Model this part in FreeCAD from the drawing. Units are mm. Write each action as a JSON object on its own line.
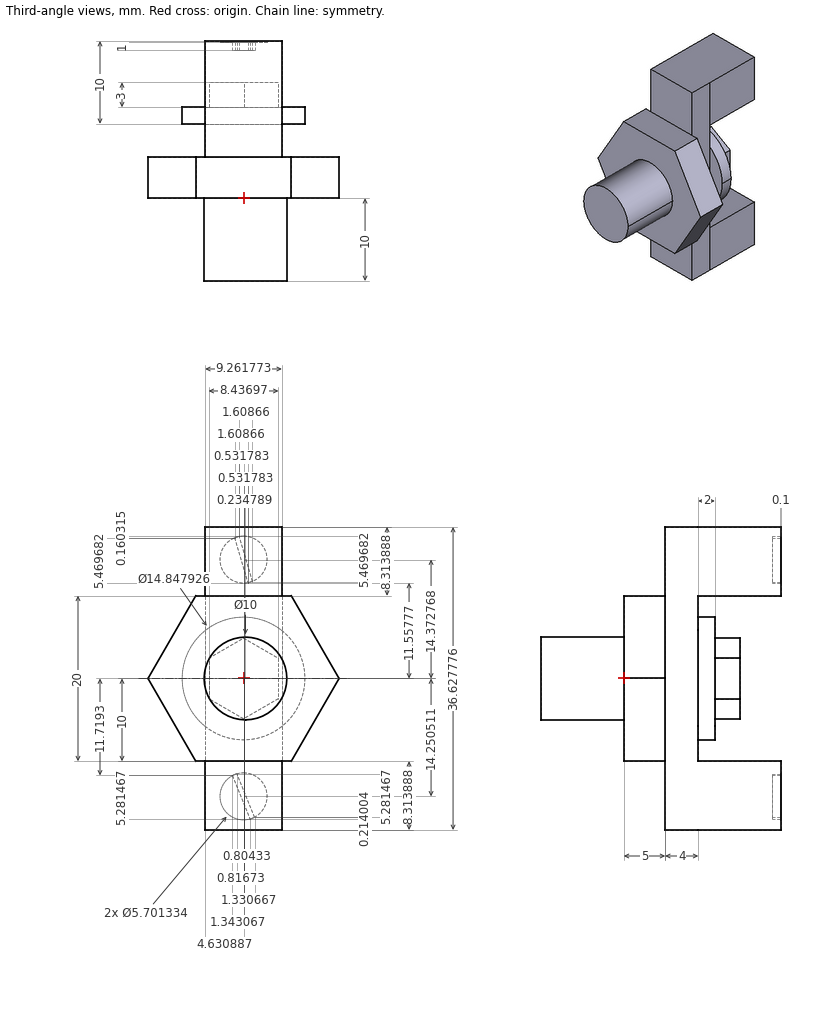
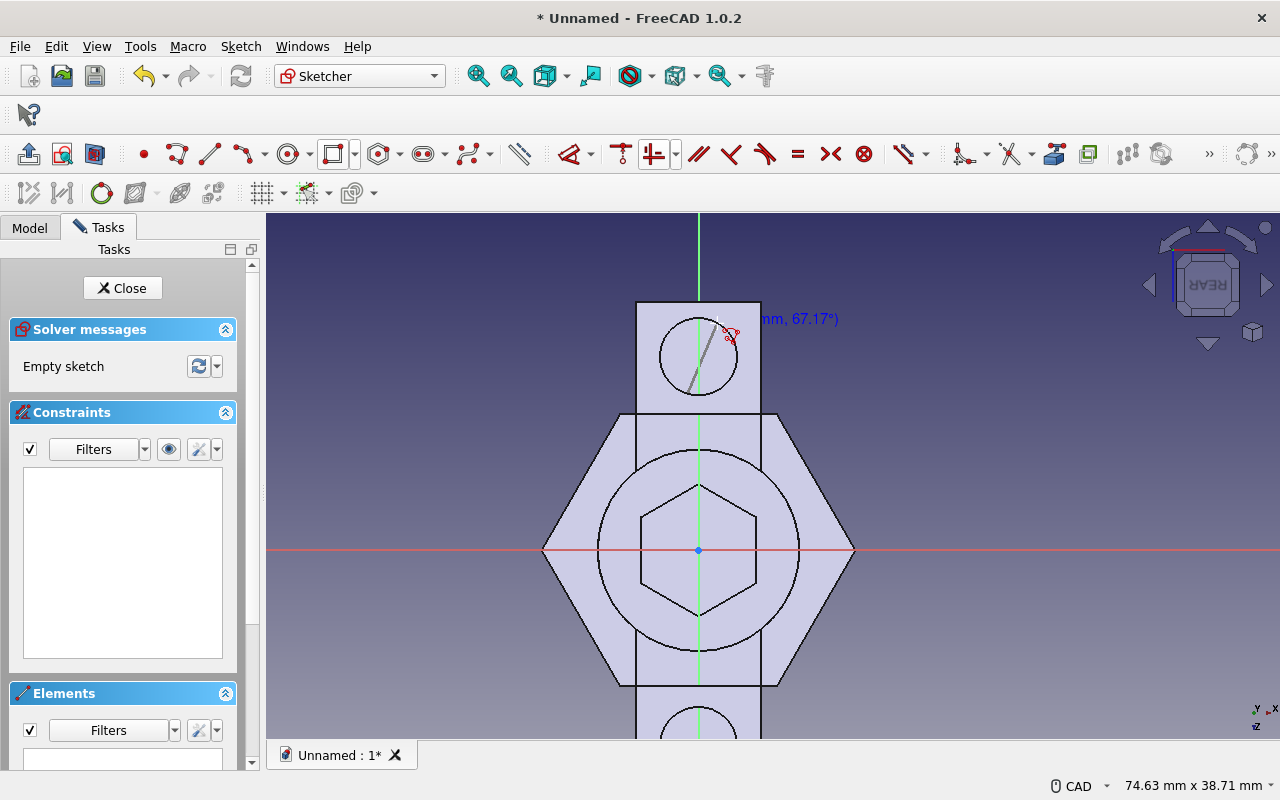
{"action": "left_click", "coordinate": [717, 322]}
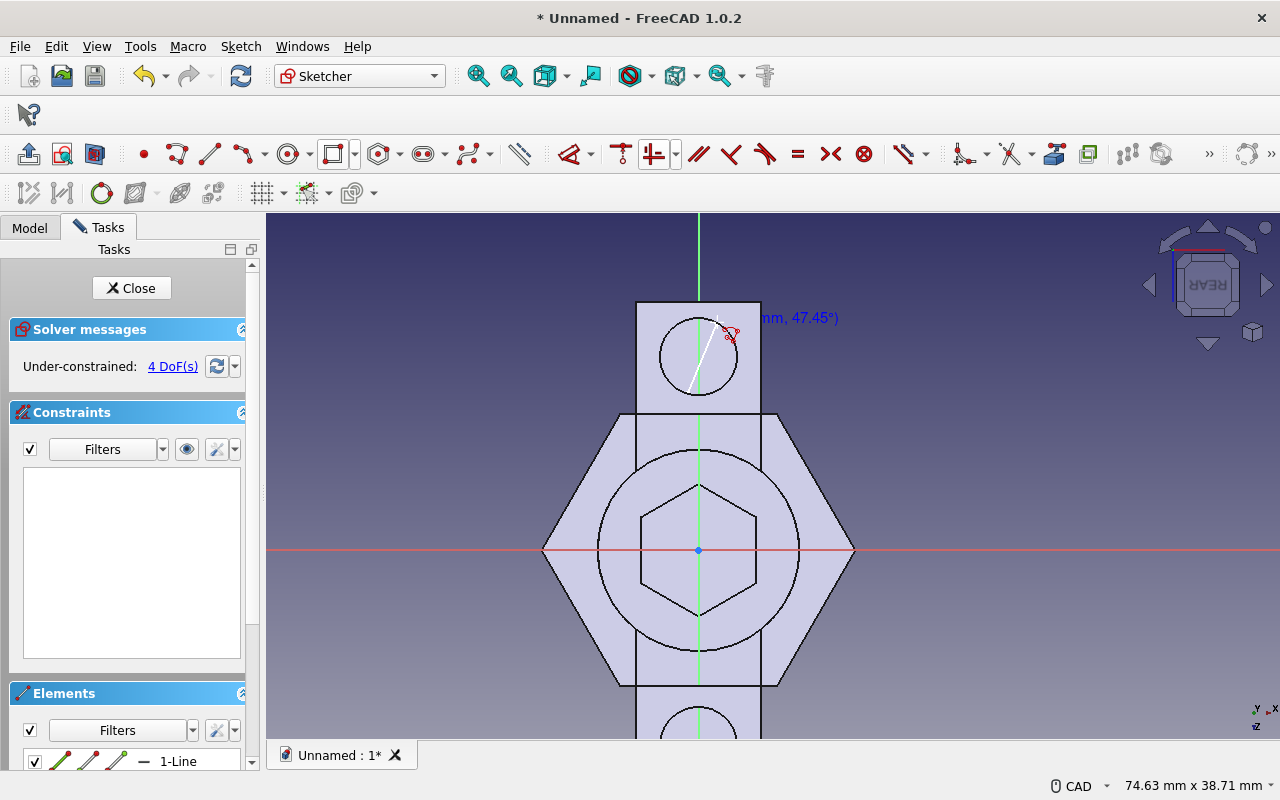
{"action": "scroll", "coordinate": [709, 319], "scroll_direction": "up", "scroll_amount": 4}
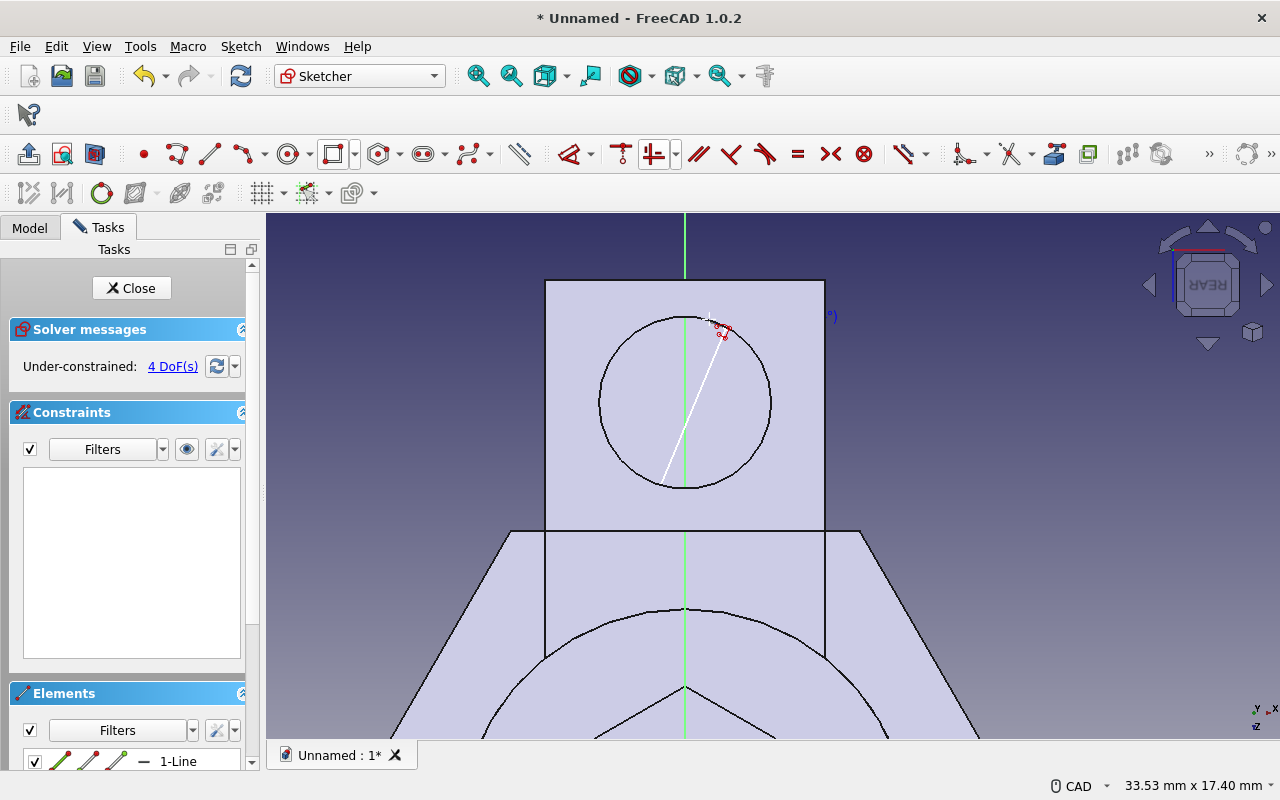
{"action": "left_click", "coordinate": [709, 320]}
{"action": "left_click", "coordinate": [645, 479]}
{"action": "left_click", "coordinate": [660, 487]}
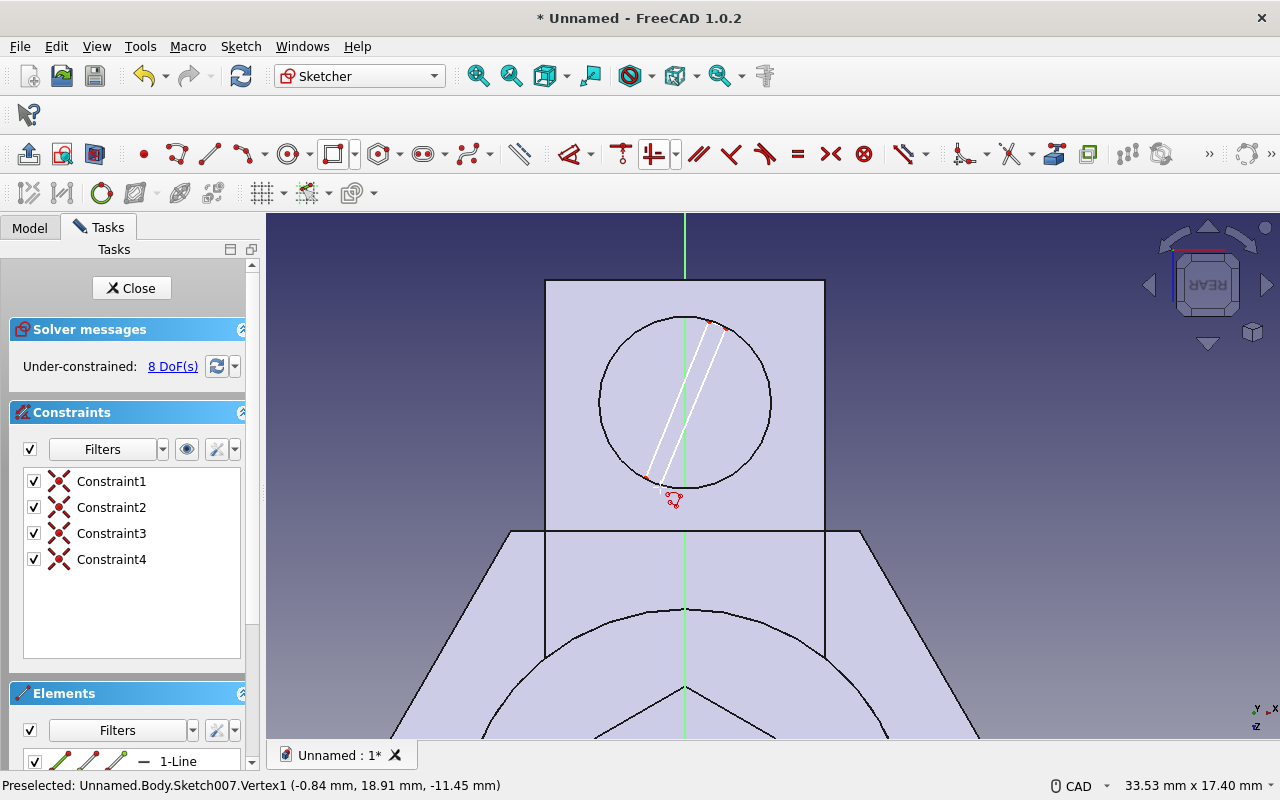
{"action": "scroll", "coordinate": [713, 321], "scroll_direction": "down", "scroll_amount": 6}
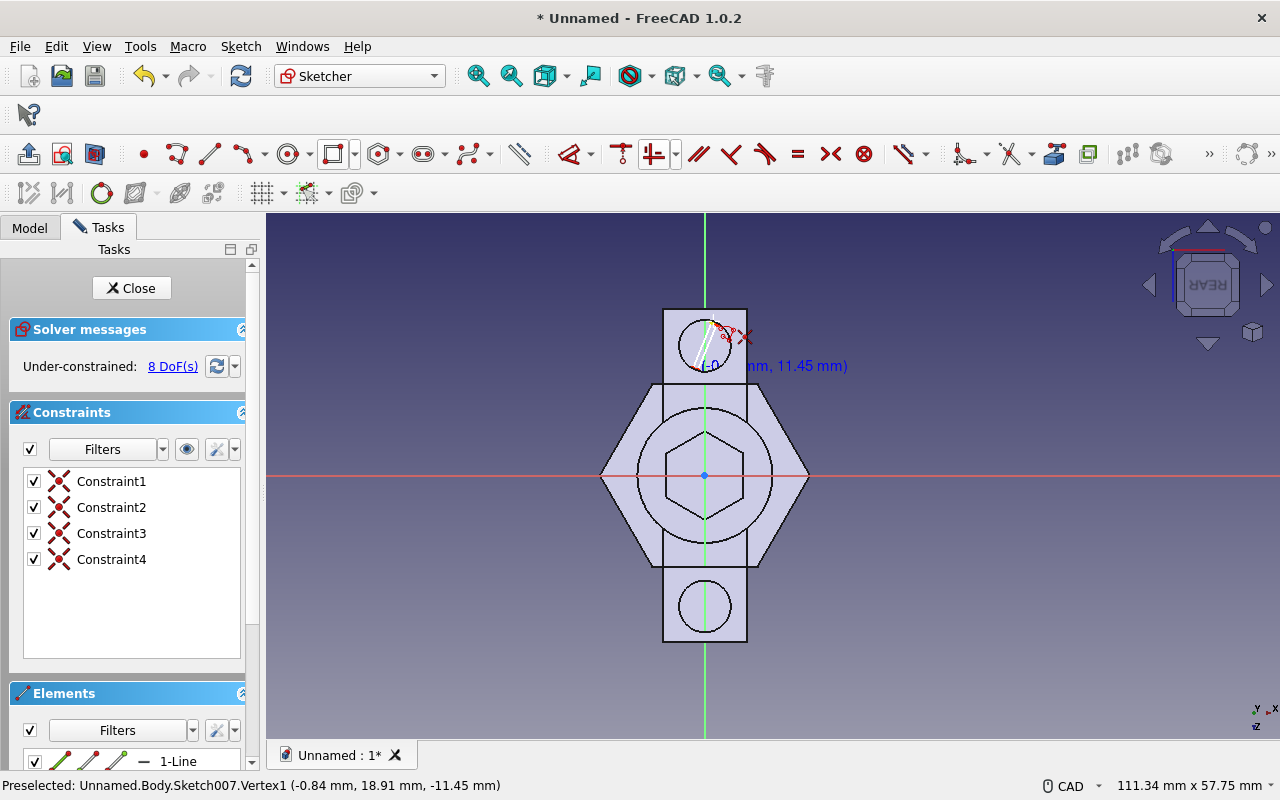
{"action": "scroll", "coordinate": [710, 581], "scroll_direction": "up", "scroll_amount": 6}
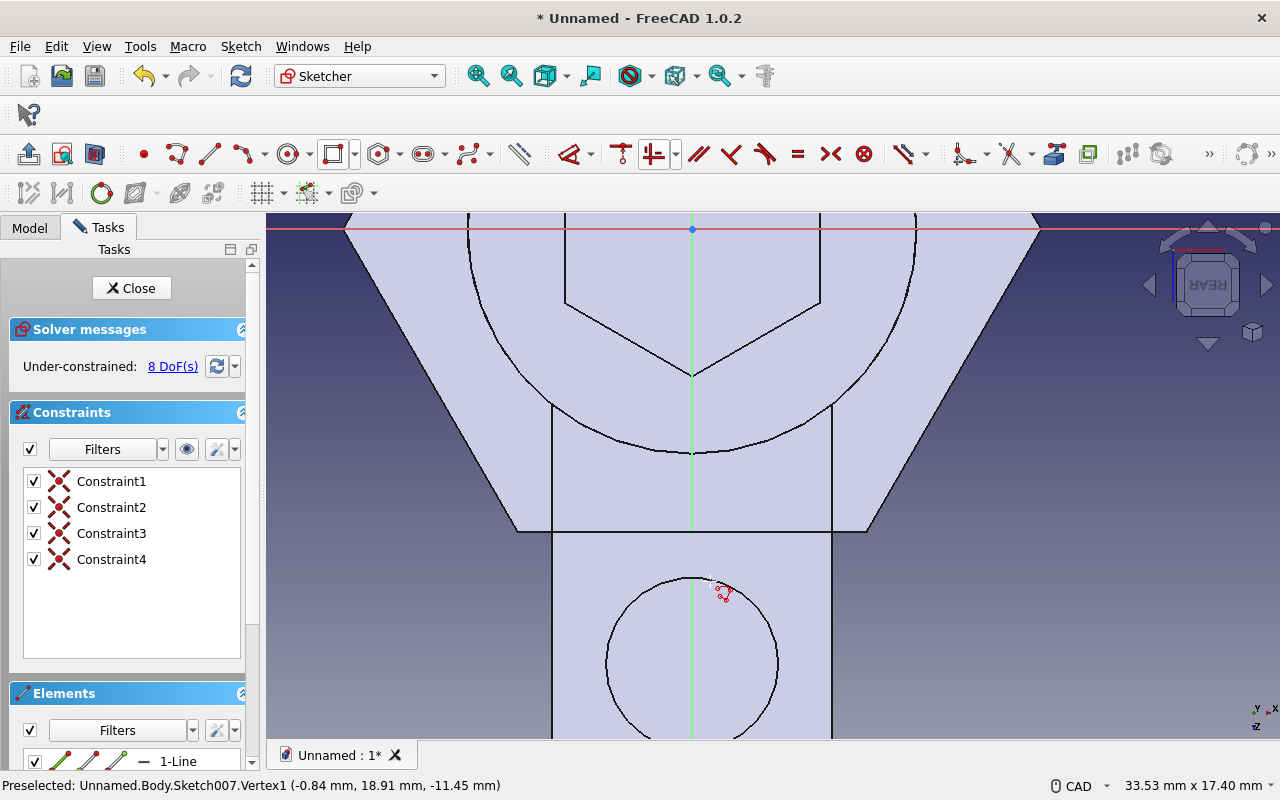
{"action": "left_click", "coordinate": [708, 579]}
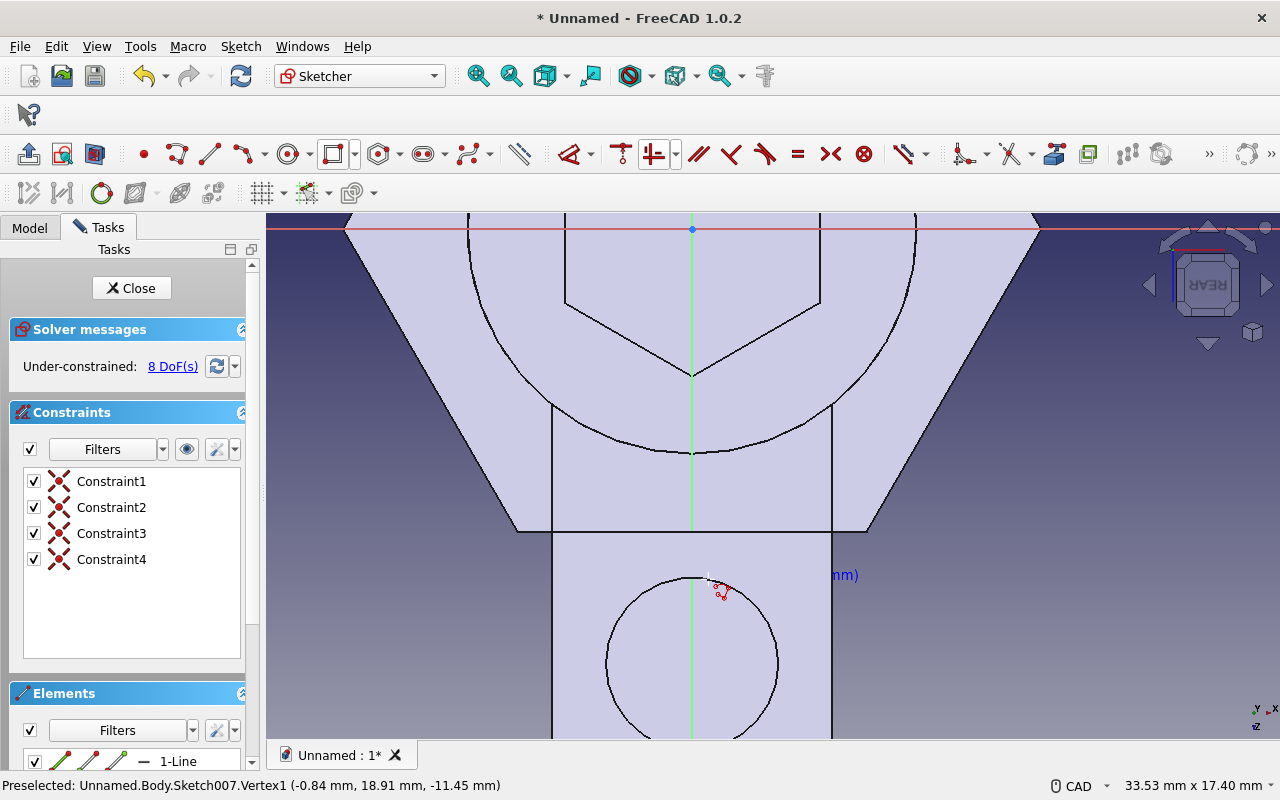
{"action": "scroll", "coordinate": [710, 581], "scroll_direction": "down", "scroll_amount": 6}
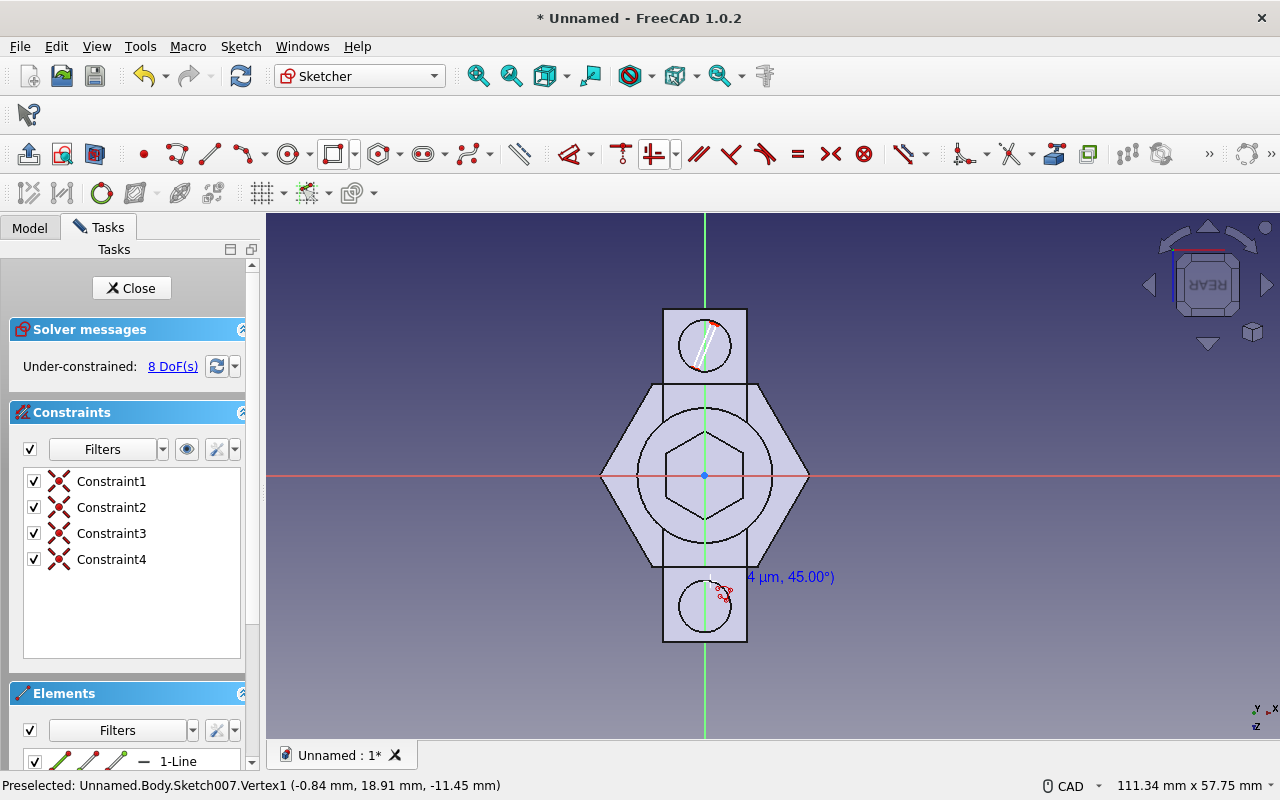
{"action": "scroll", "coordinate": [695, 631], "scroll_direction": "up", "scroll_amount": 3}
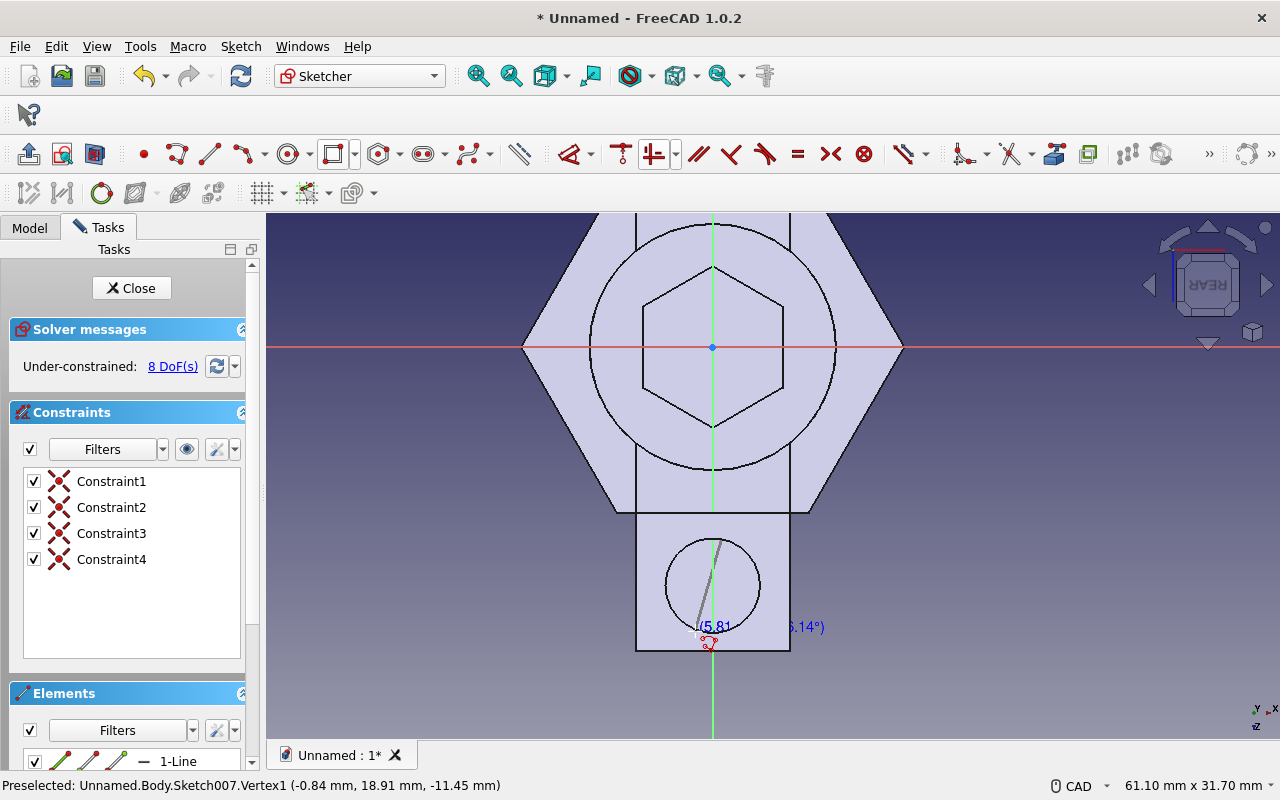
{"action": "left_click", "coordinate": [695, 630]}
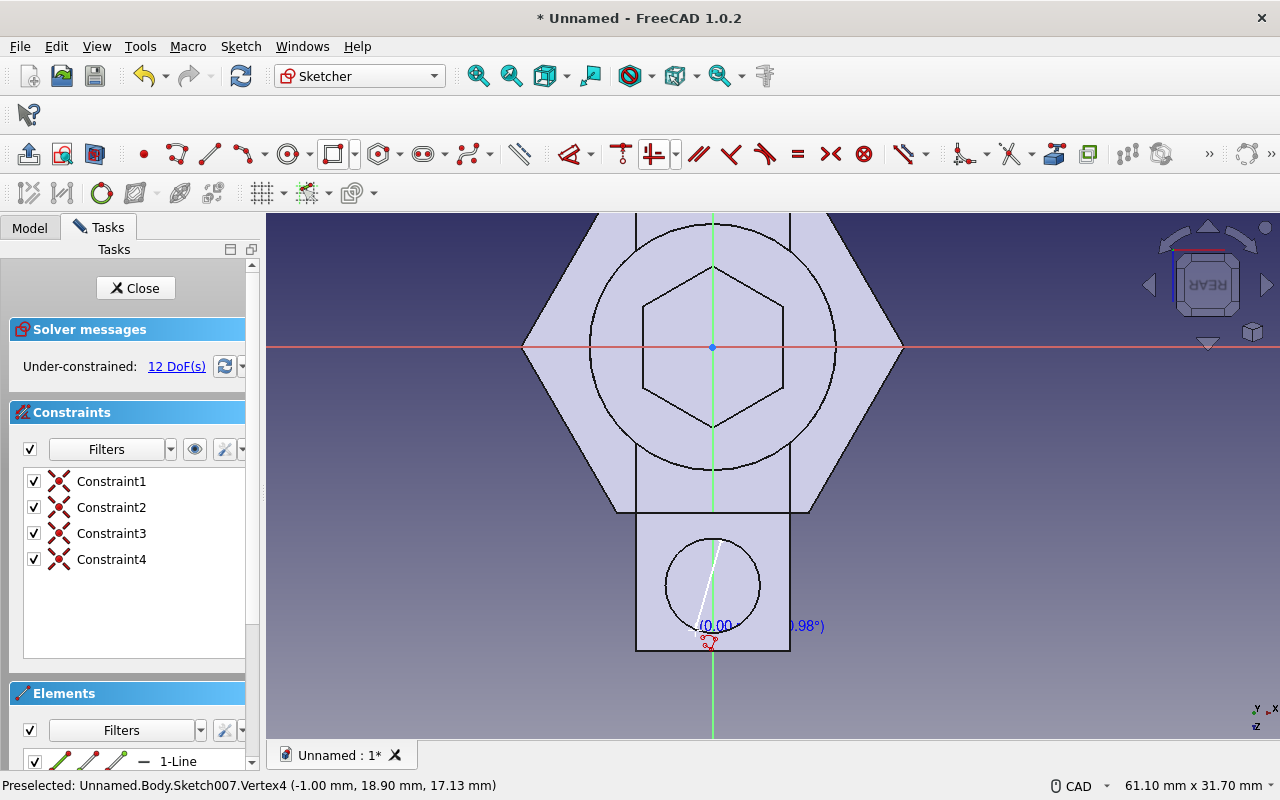
{"action": "scroll", "coordinate": [704, 632], "scroll_direction": "up", "scroll_amount": 3}